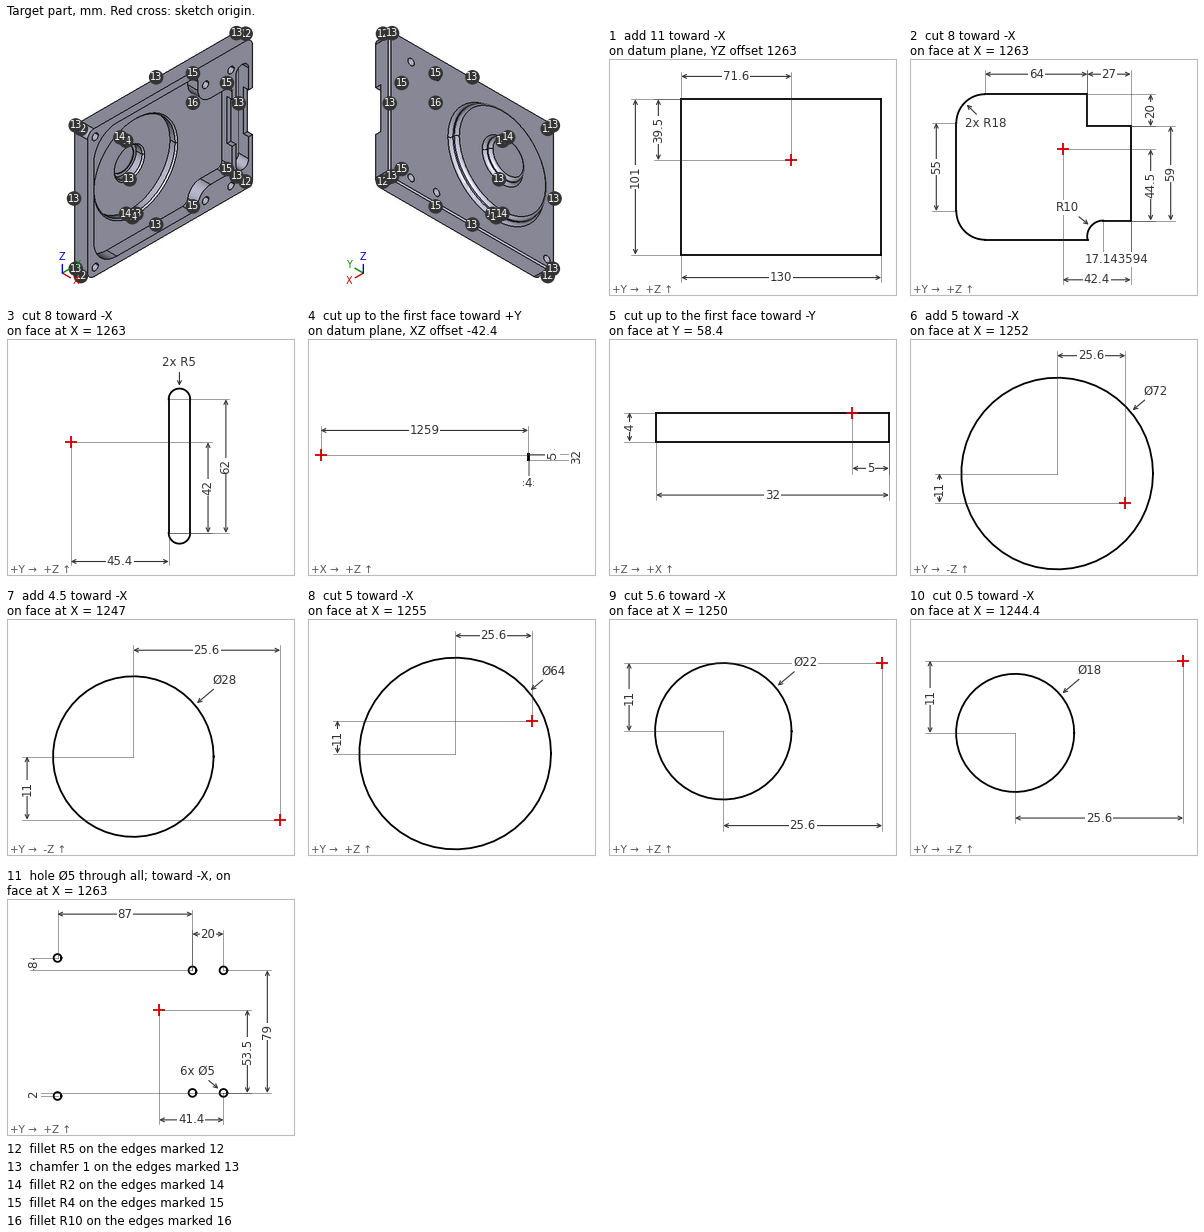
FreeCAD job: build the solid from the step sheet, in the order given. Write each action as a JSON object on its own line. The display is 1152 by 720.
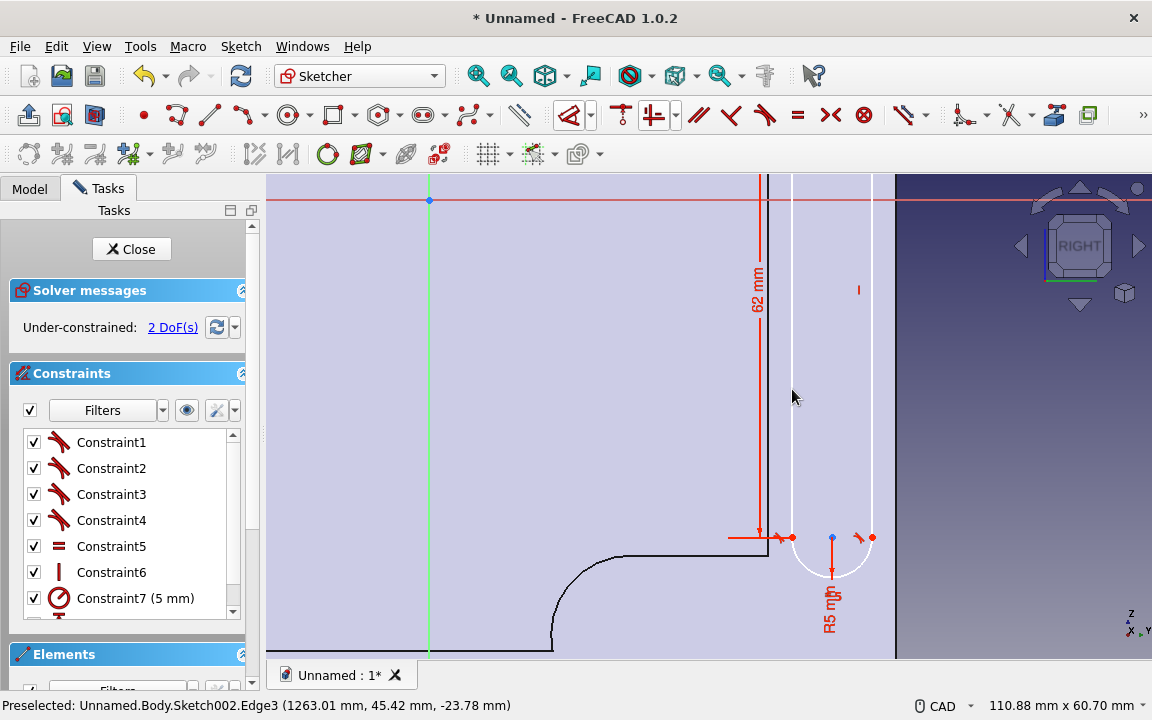
{"action": "left_click", "coordinate": [792, 538]}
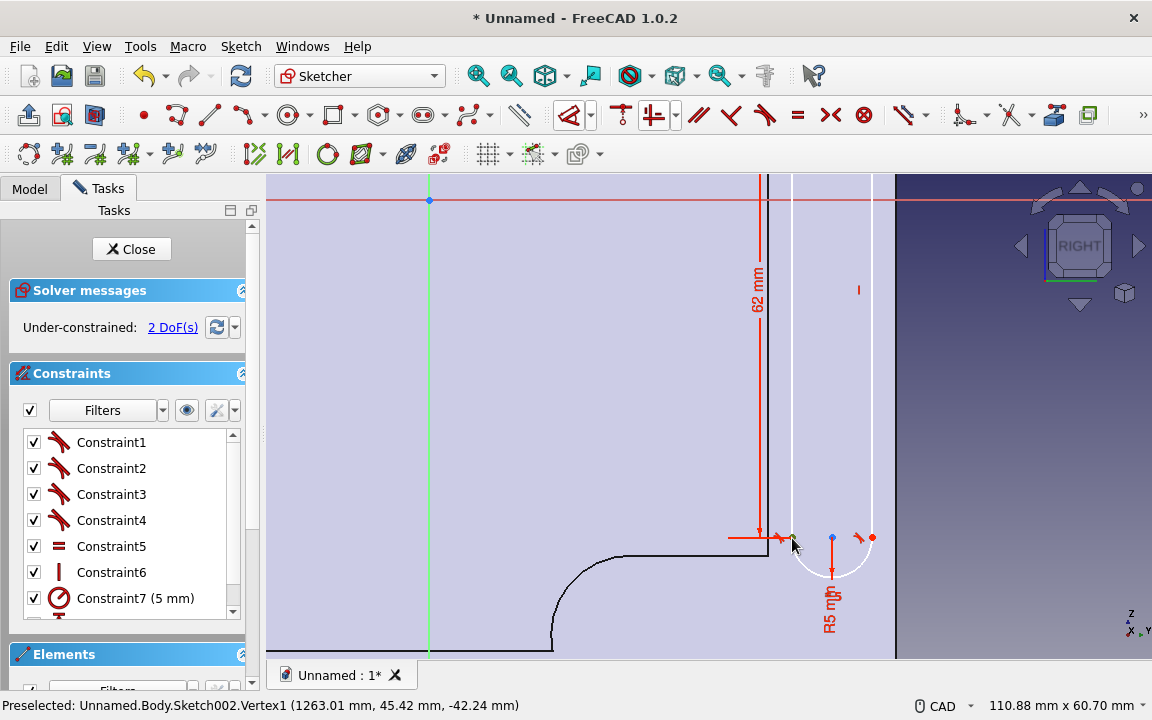
{"action": "left_click", "coordinate": [590, 116]}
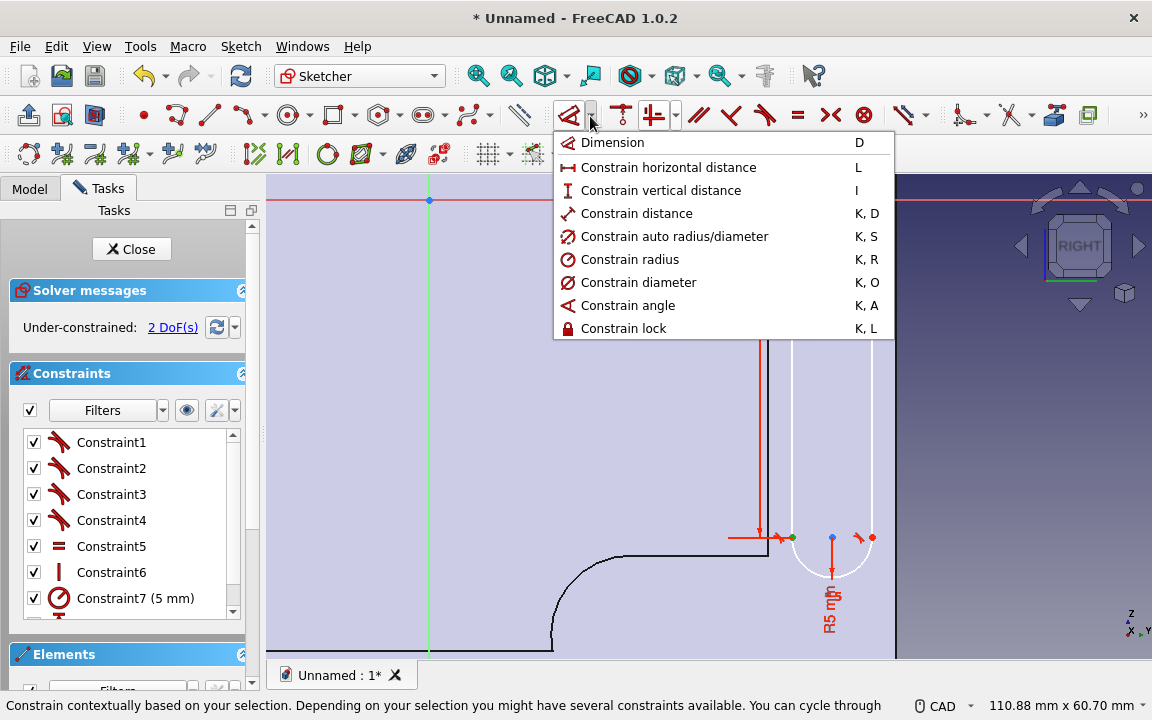
{"action": "left_click", "coordinate": [724, 190]}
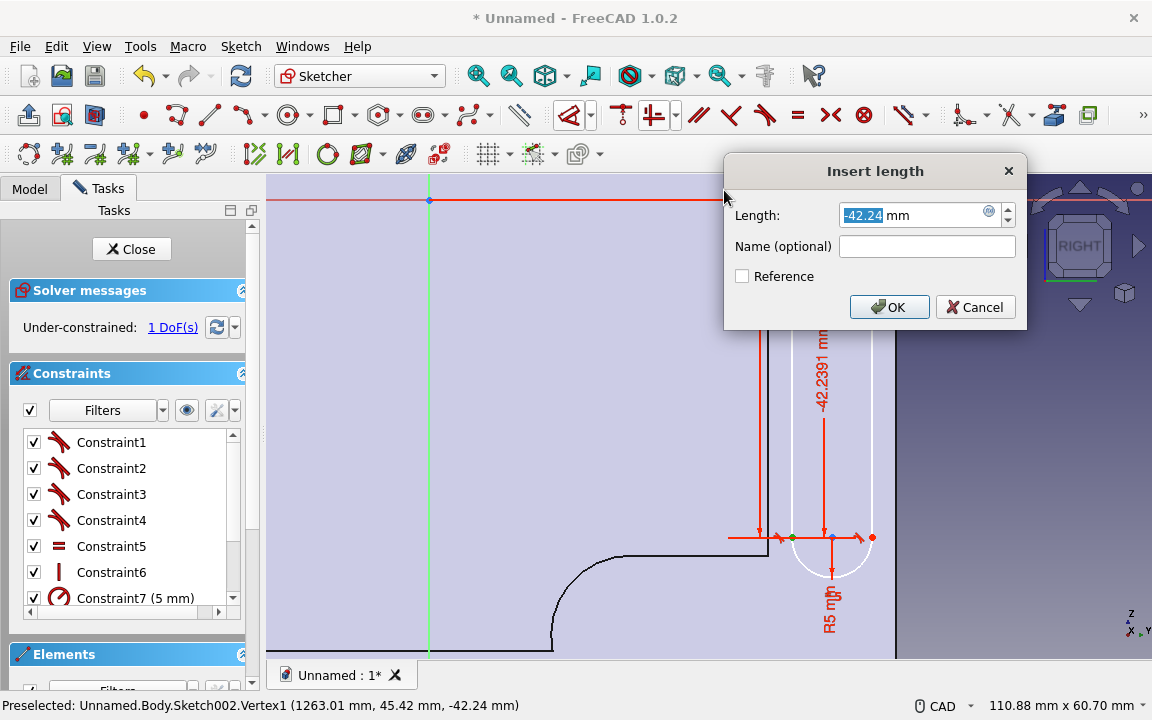
{"action": "type", "text": "-42"}
{"action": "key", "text": "Return"}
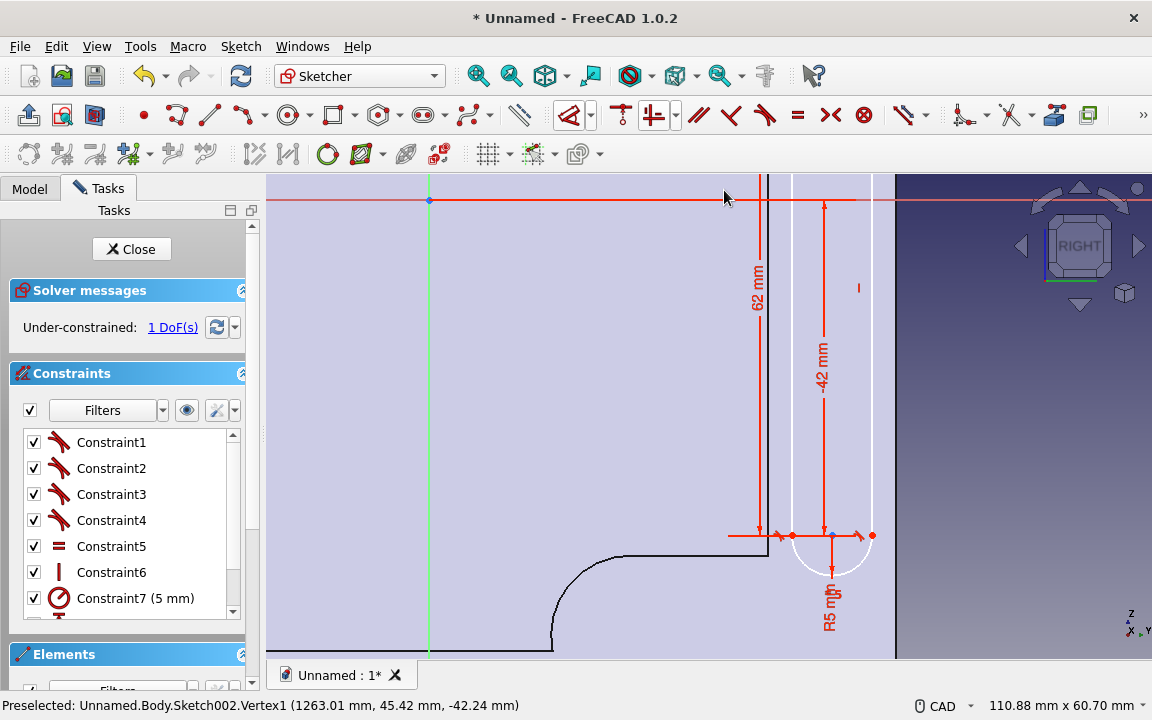
{"action": "left_click", "coordinate": [792, 536]}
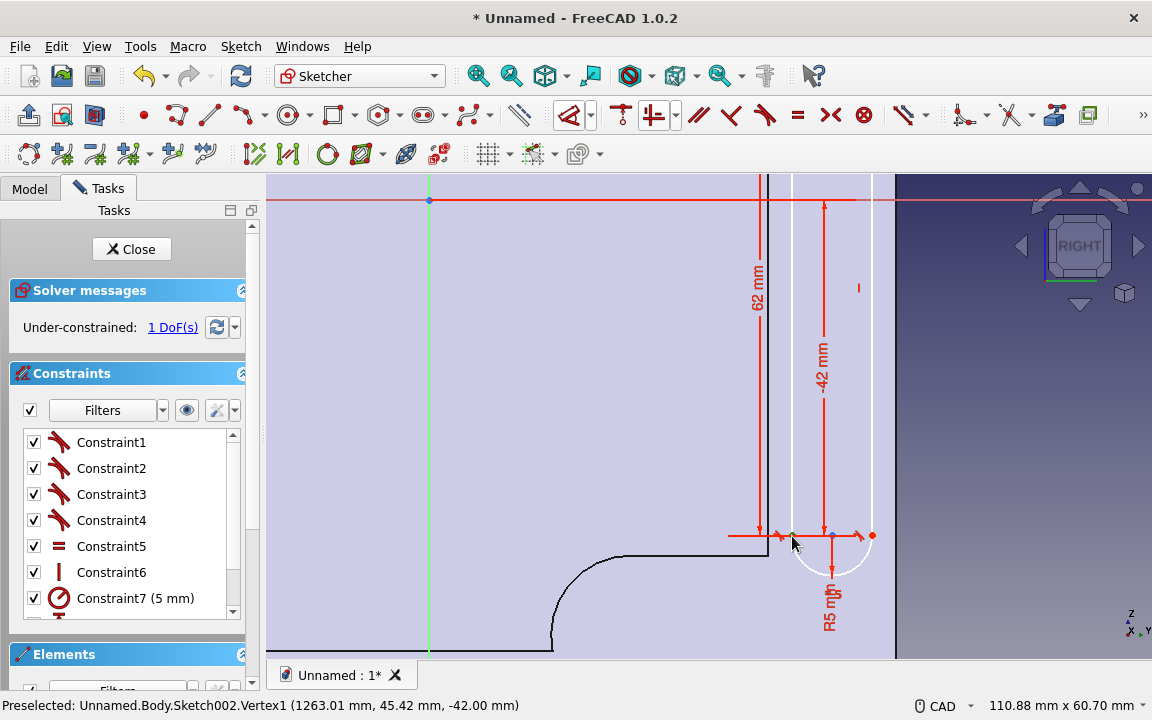
{"action": "key", "text": "l"}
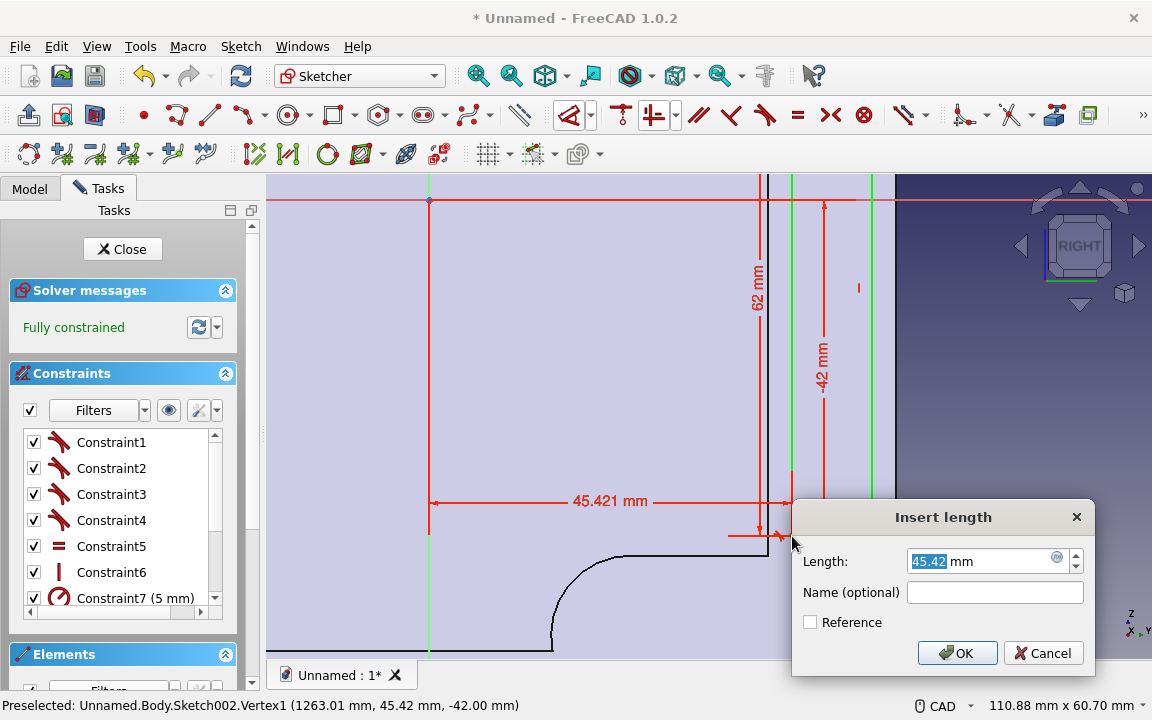
{"action": "type", "text": "45.4"}
{"action": "key", "text": "Return"}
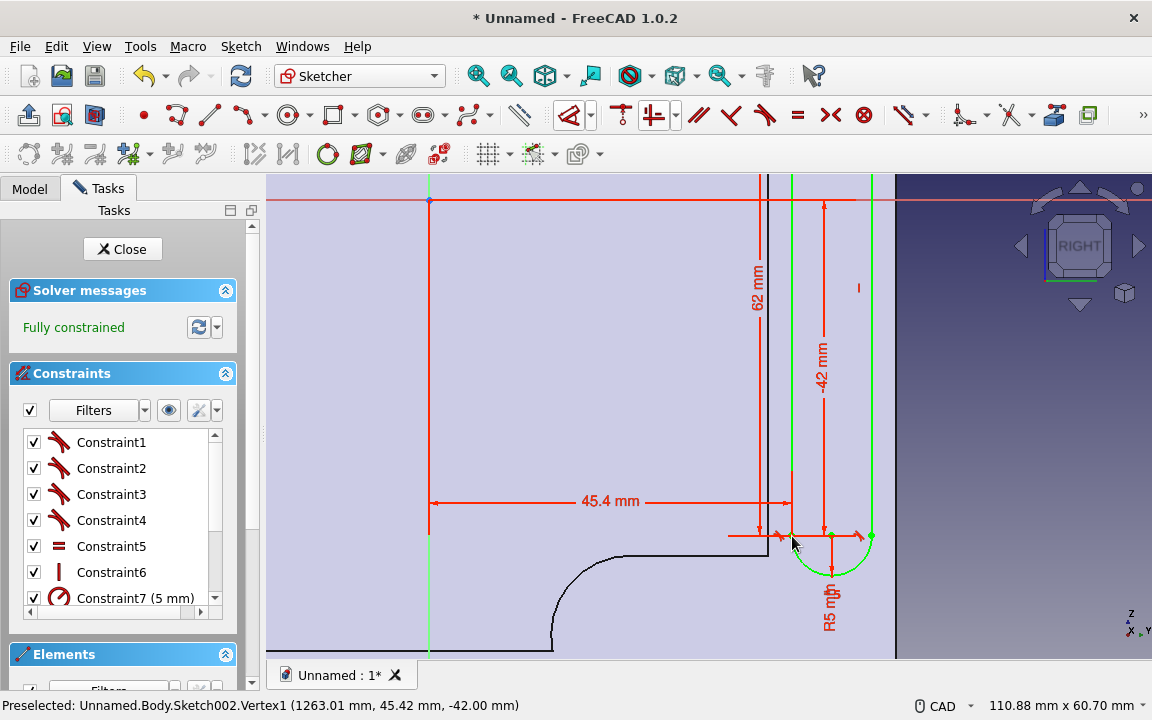
{"action": "left_click", "coordinate": [123, 249]}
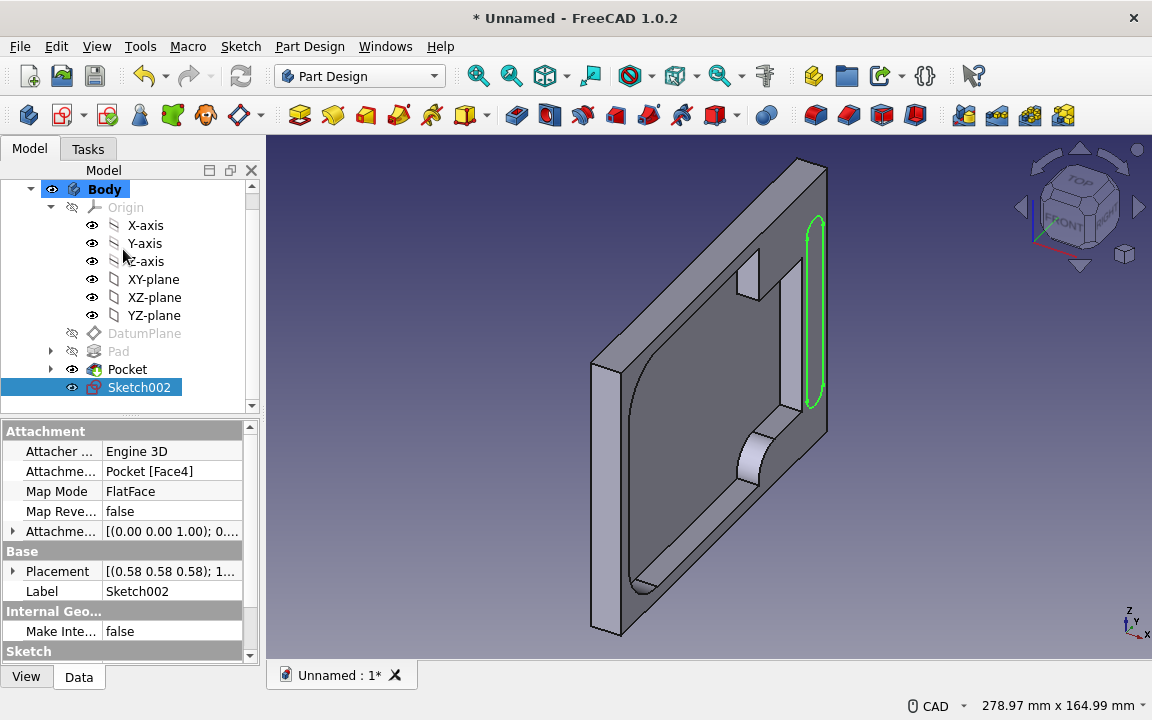
{"action": "left_click", "coordinate": [517, 116]}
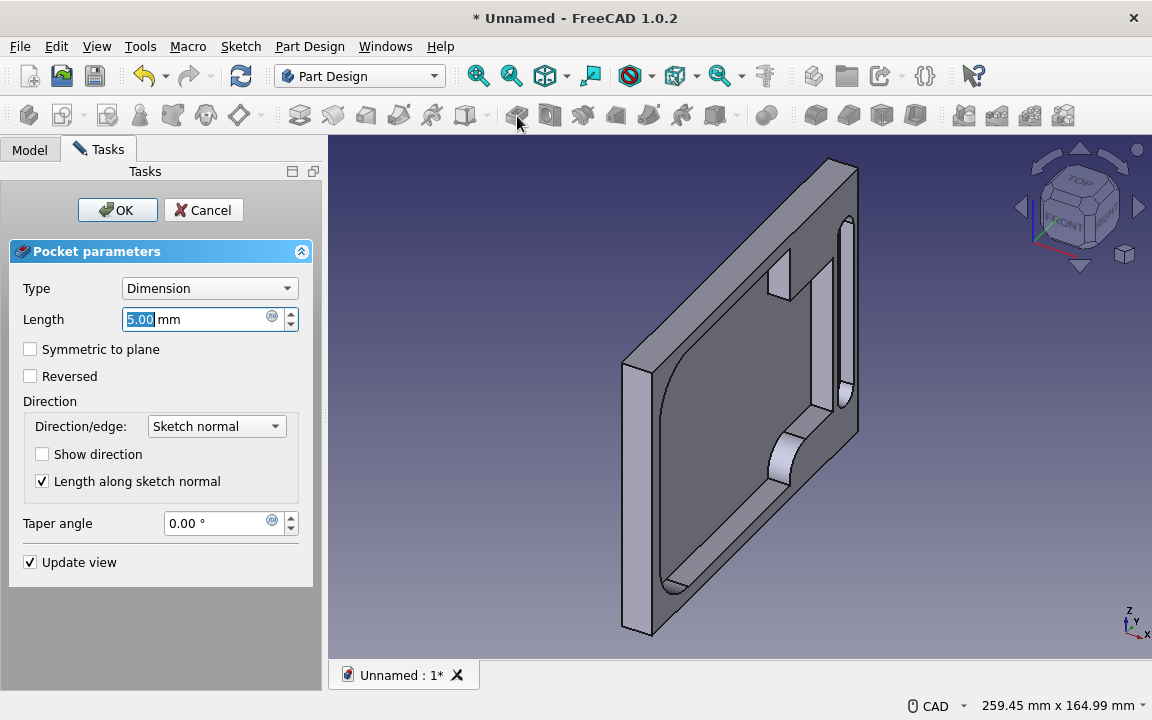
{"action": "type", "text": "8"}
{"action": "key", "text": "Tab"}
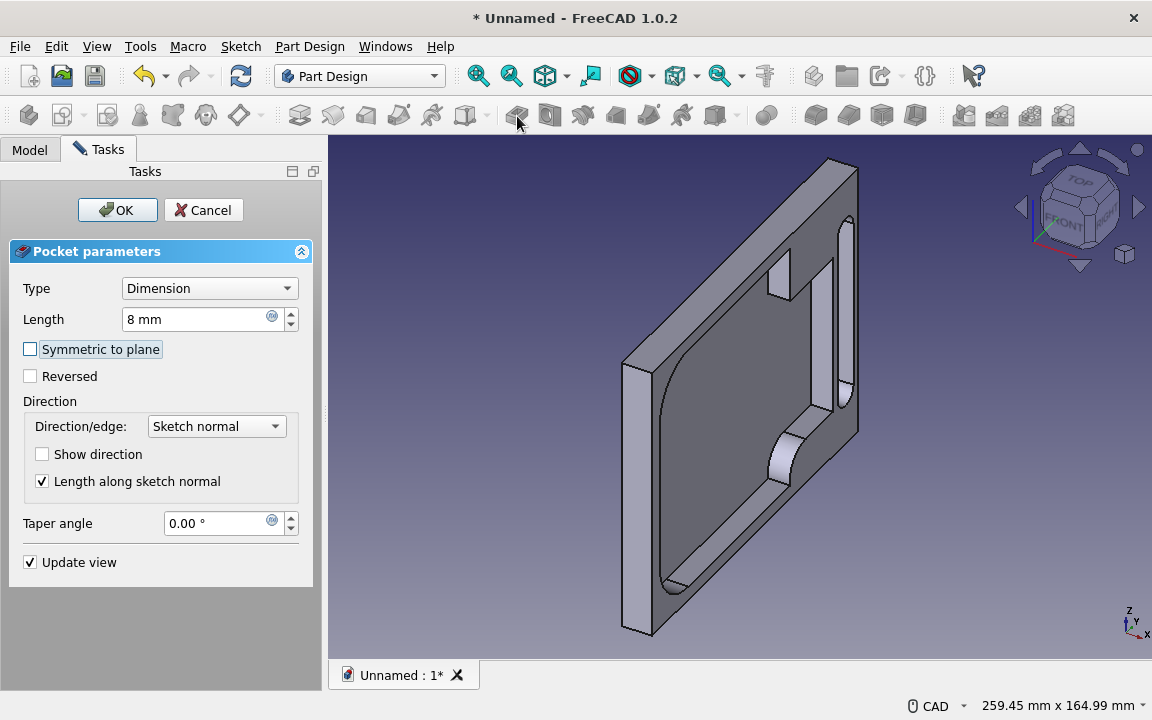
{"action": "left_click", "coordinate": [118, 210]}